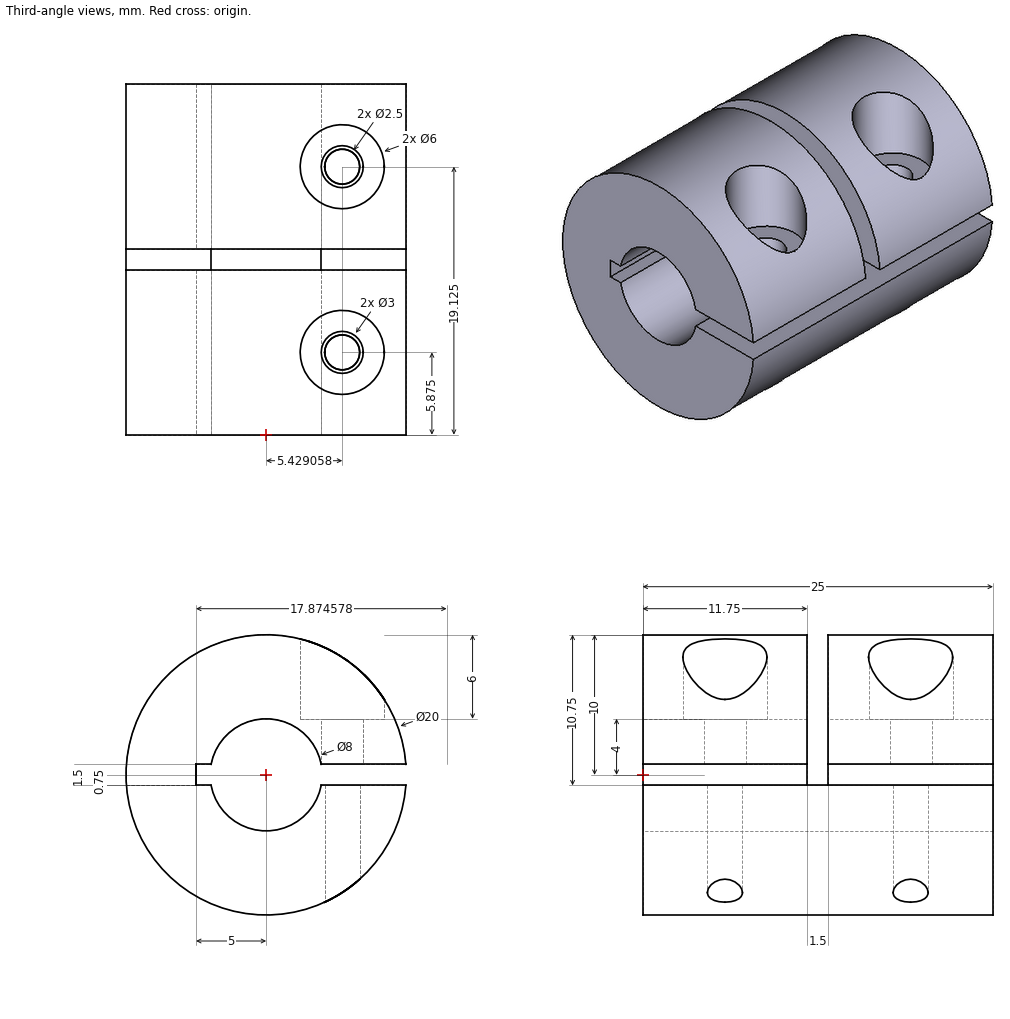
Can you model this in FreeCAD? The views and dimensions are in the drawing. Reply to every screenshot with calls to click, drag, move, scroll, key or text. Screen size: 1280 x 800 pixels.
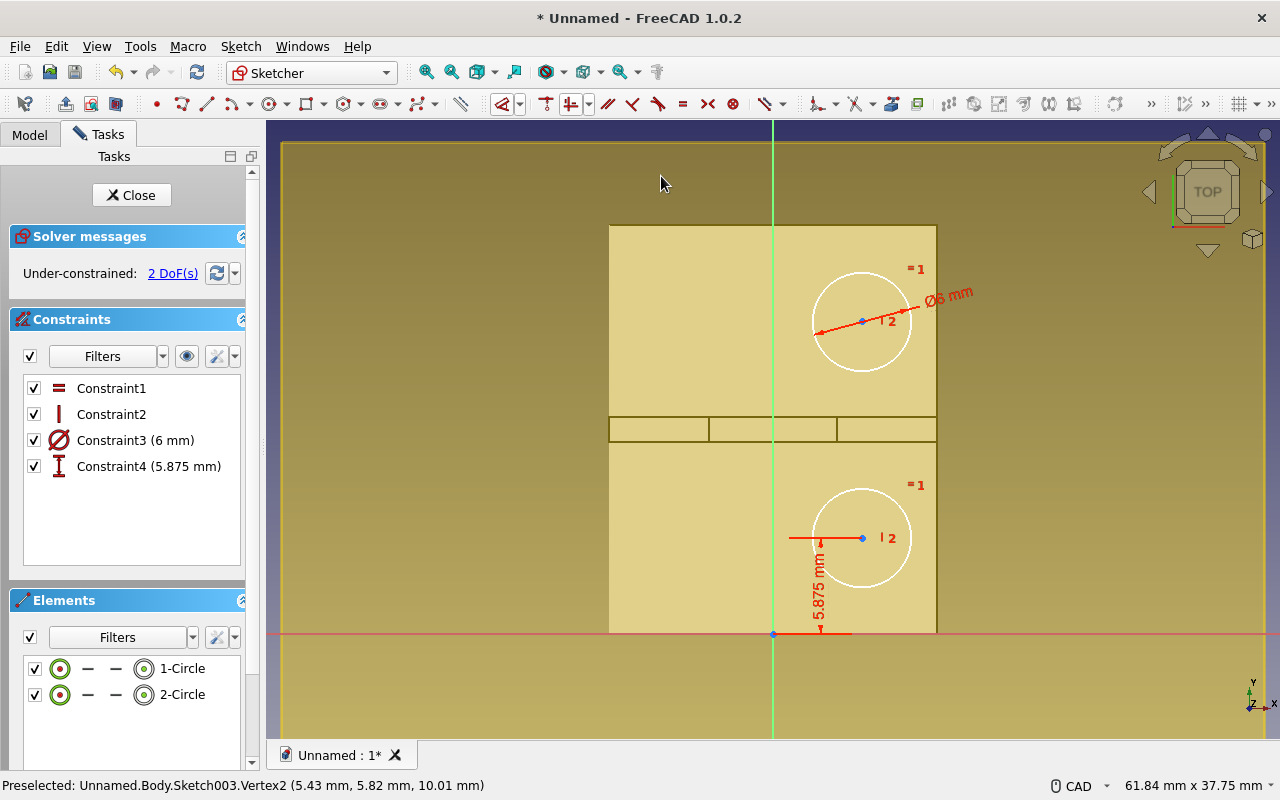
click(862, 322)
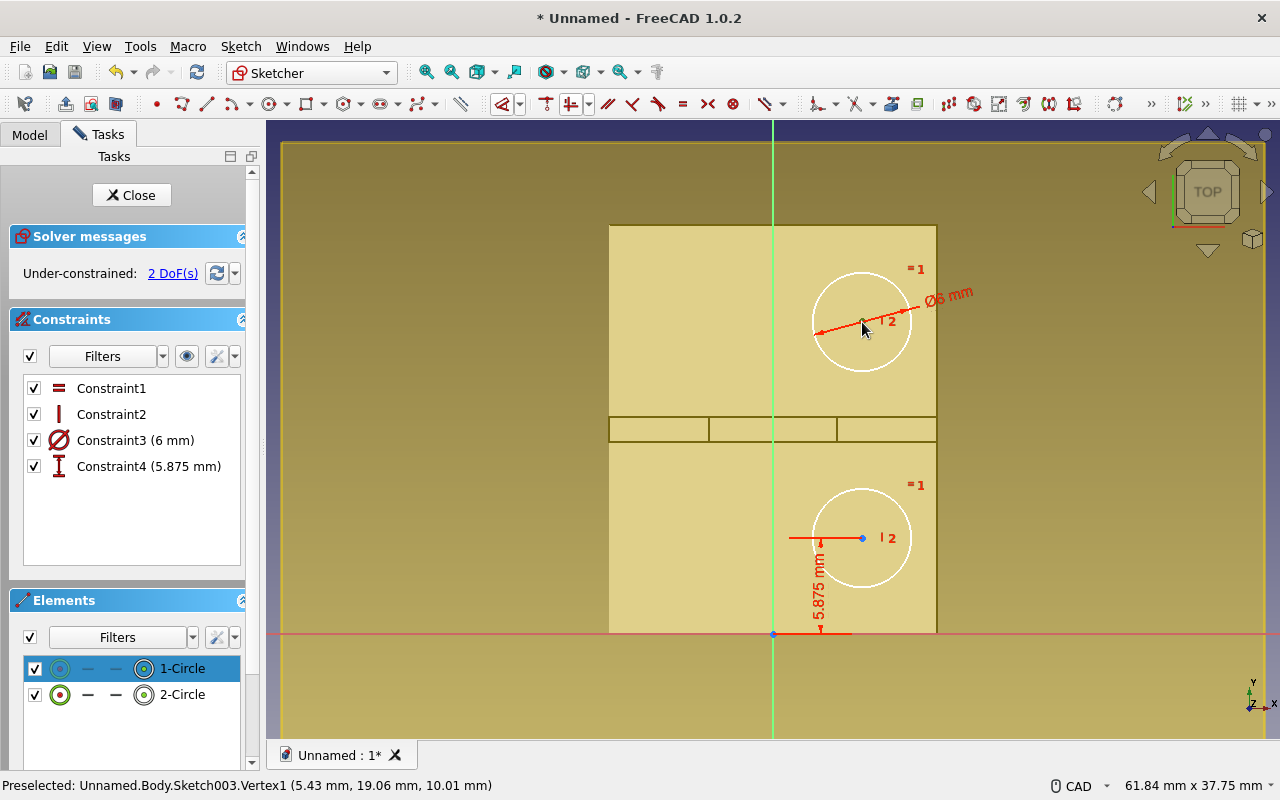
click(520, 104)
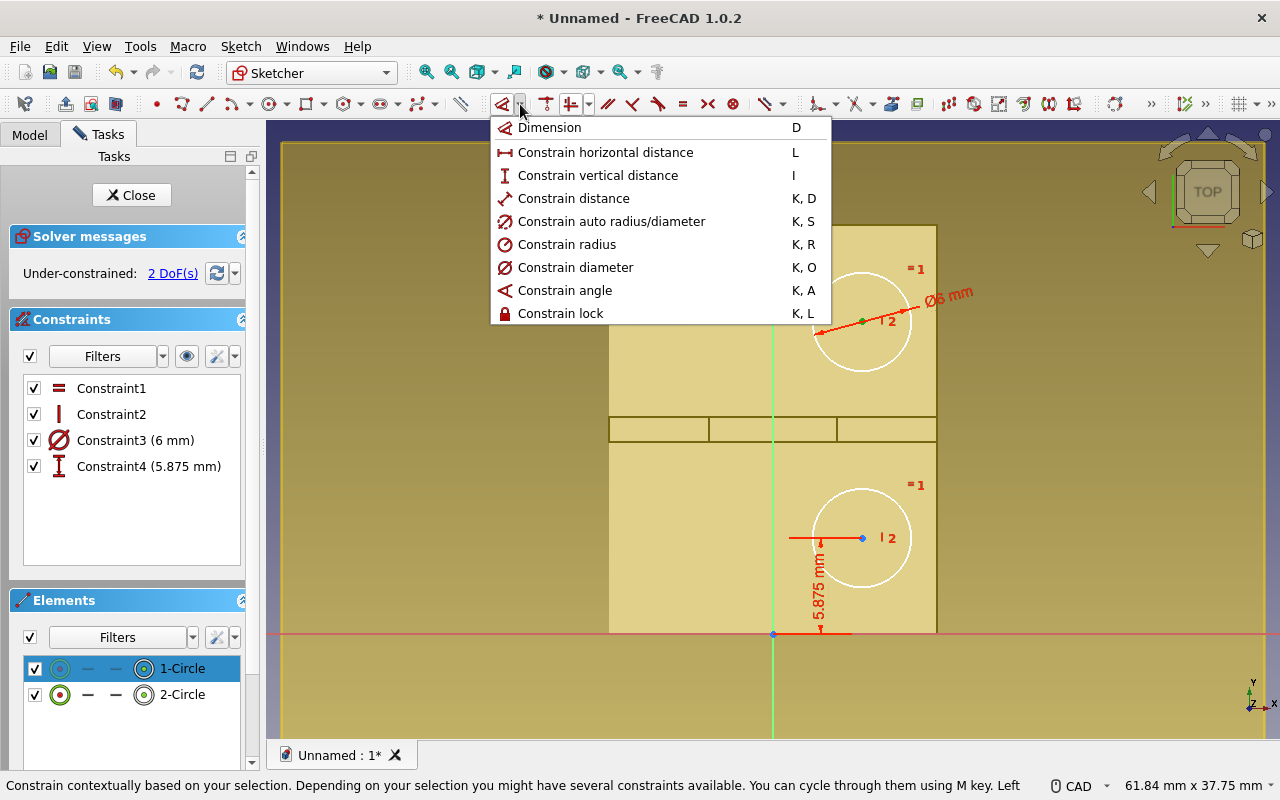
click(661, 176)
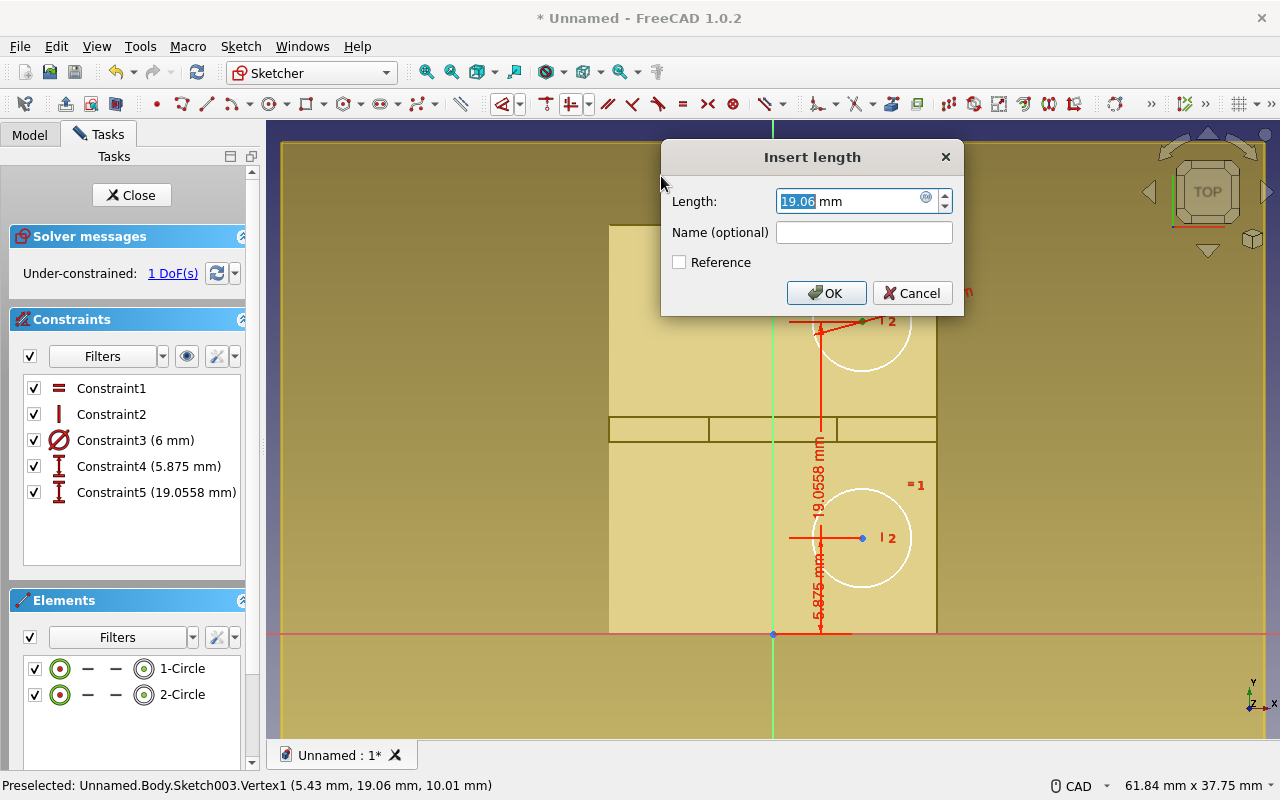
text(19.125)
key(Return)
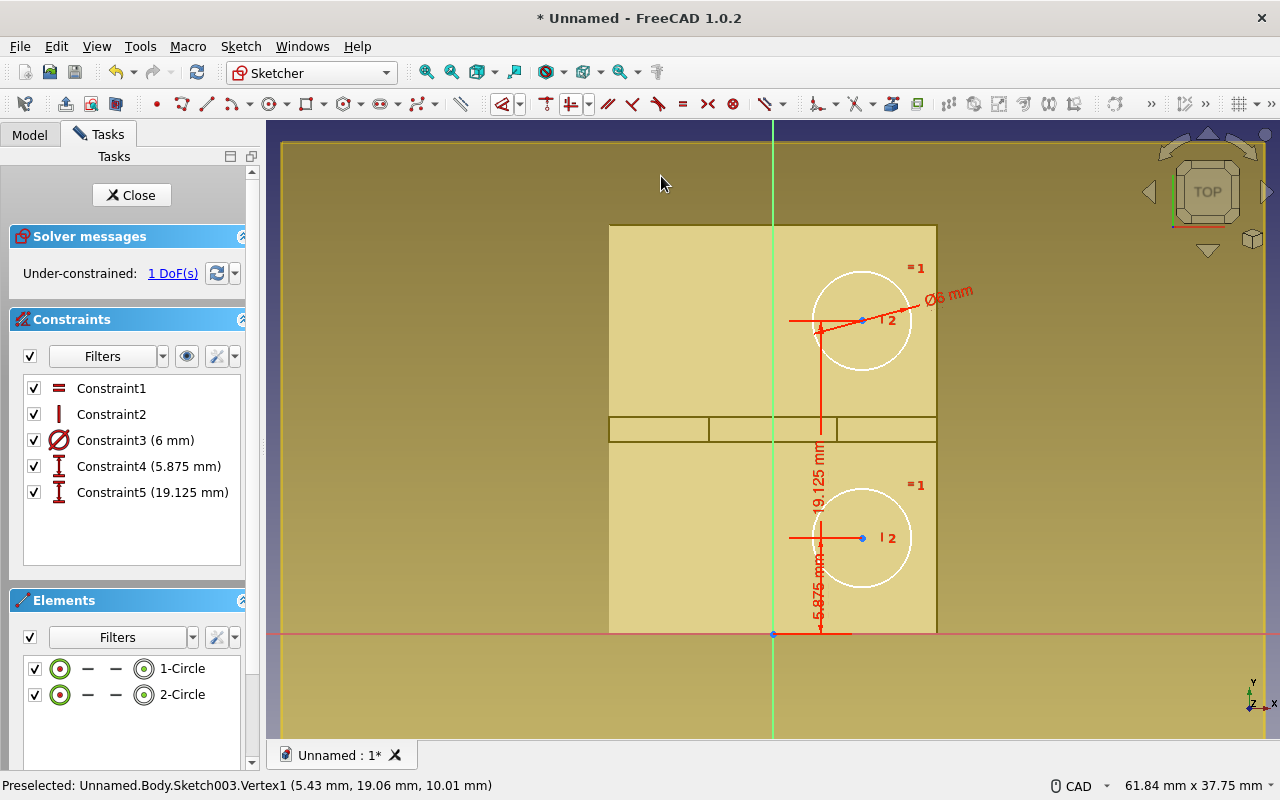
click(862, 321)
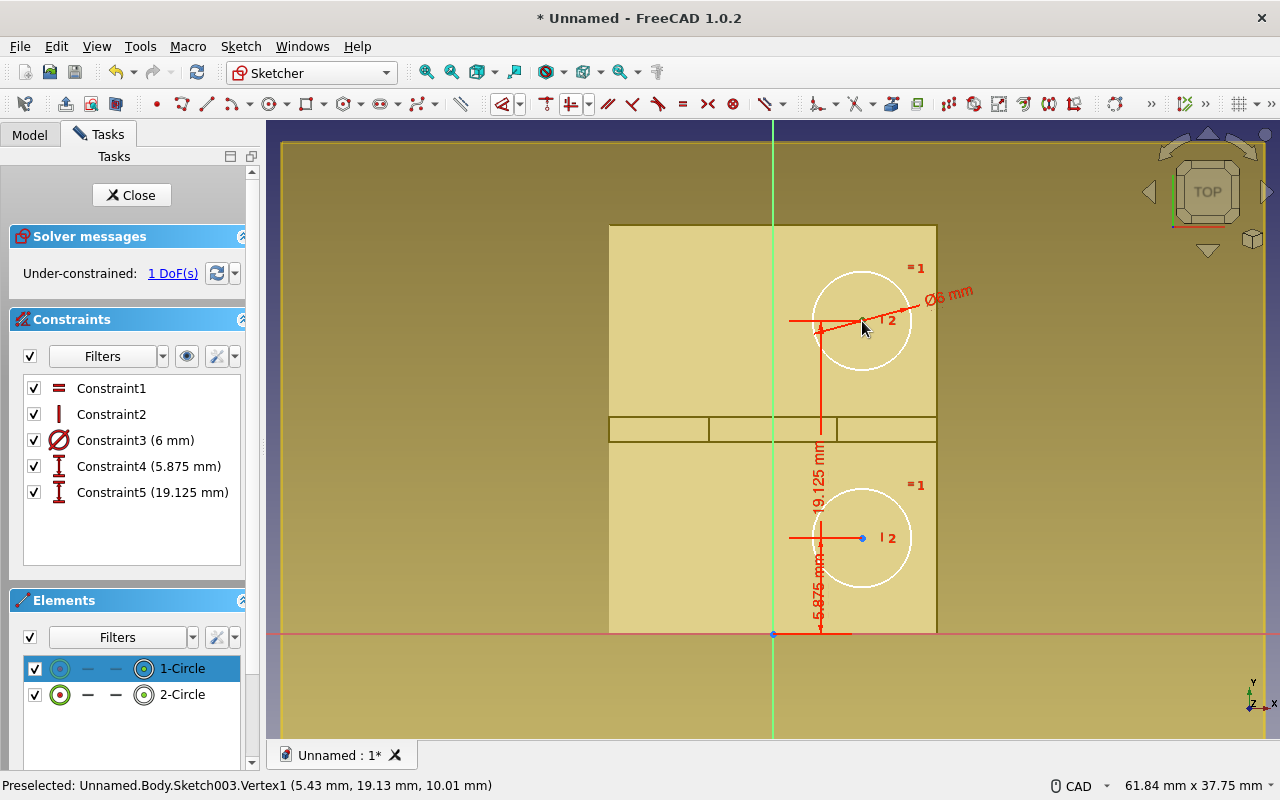
click(520, 104)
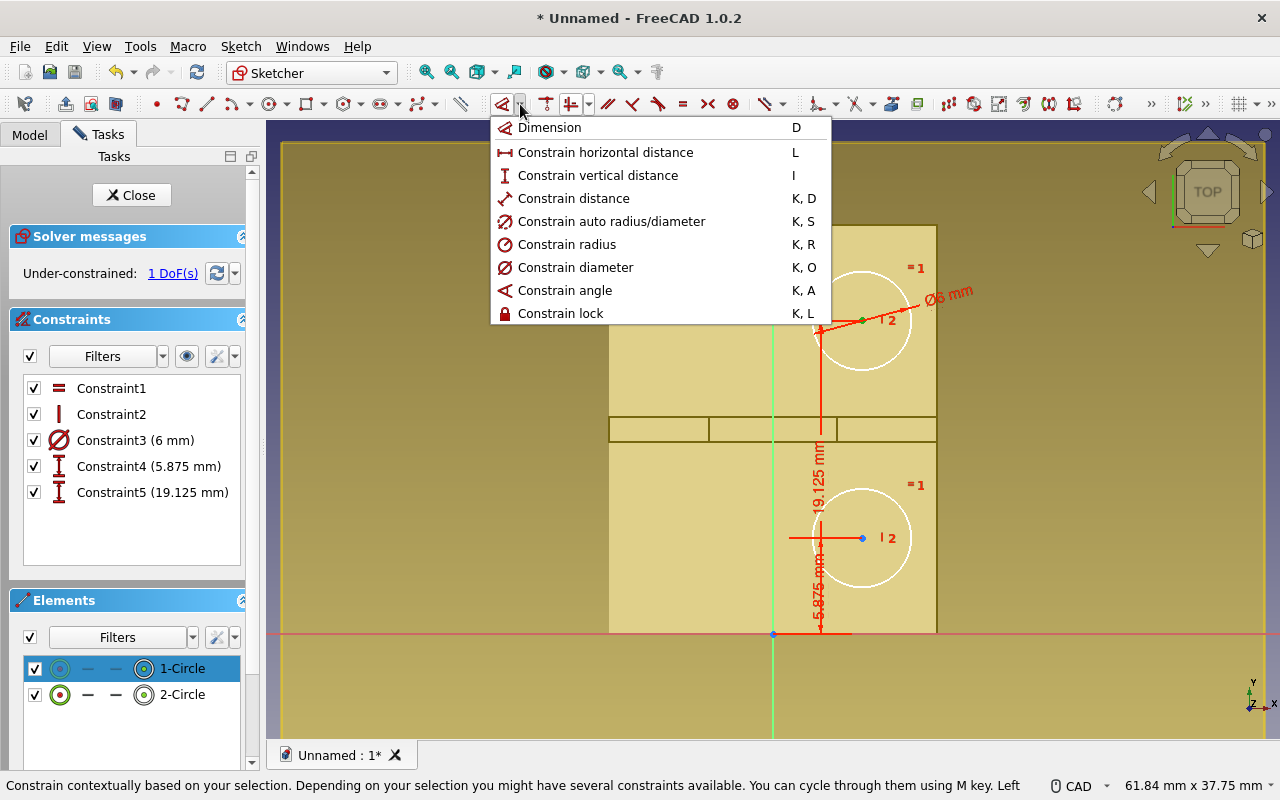
click(661, 152)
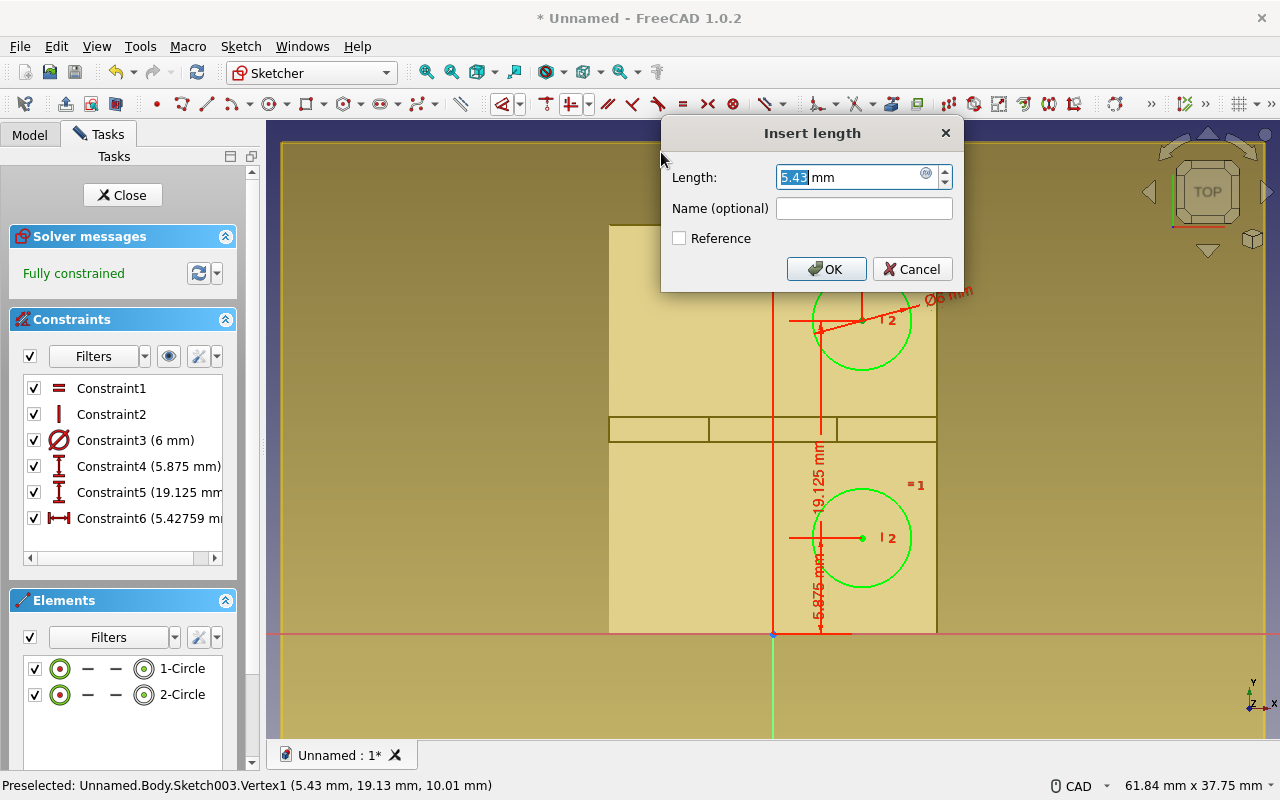
text(5.429058)
key(Return)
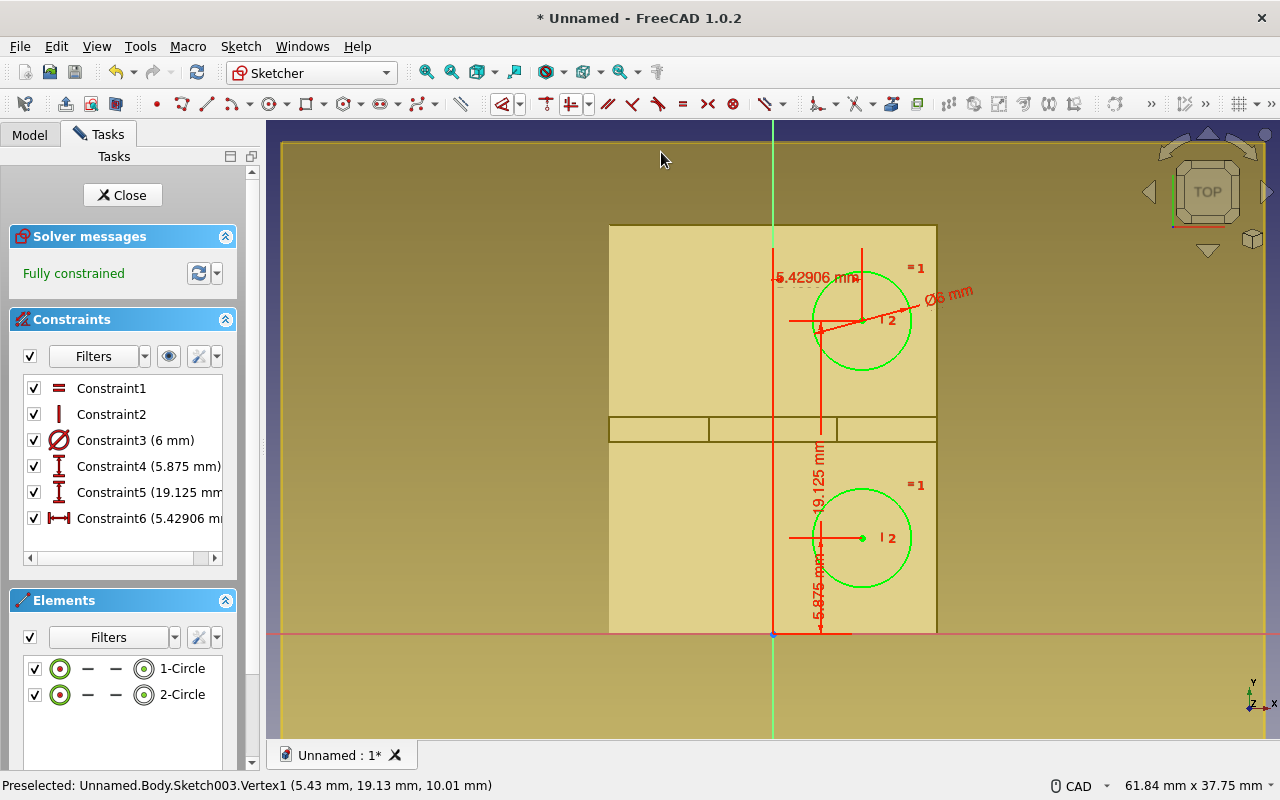
click(123, 195)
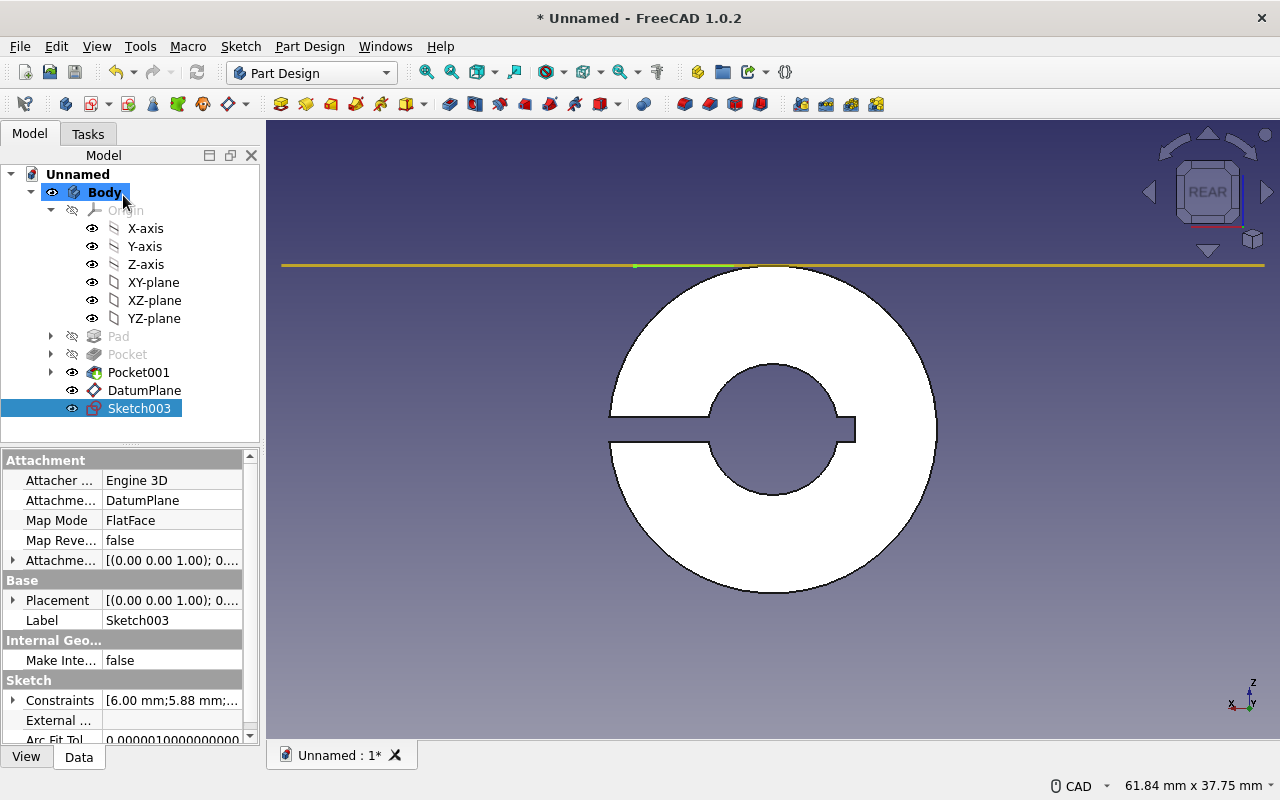
click(450, 104)